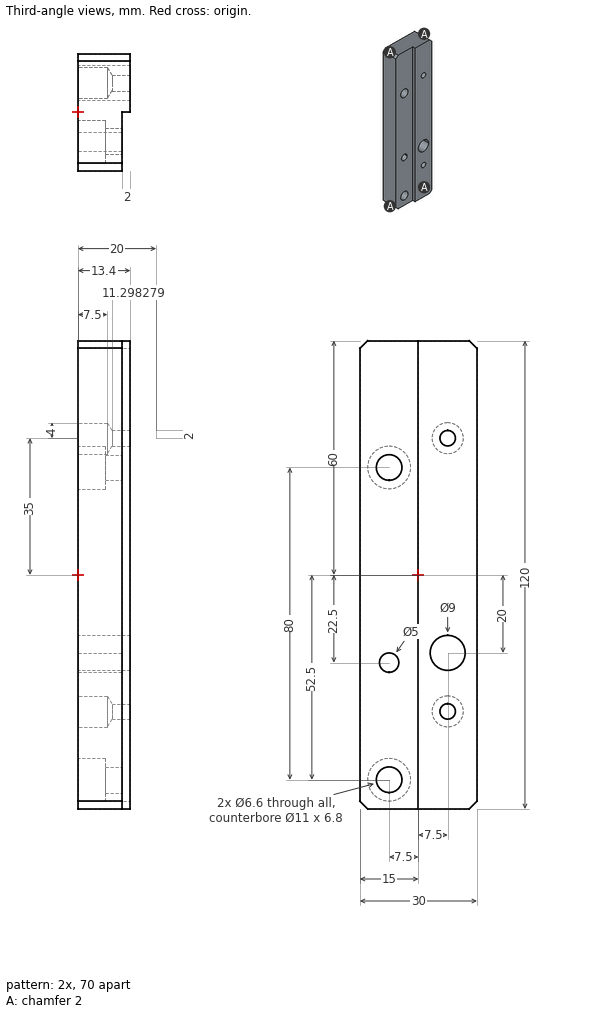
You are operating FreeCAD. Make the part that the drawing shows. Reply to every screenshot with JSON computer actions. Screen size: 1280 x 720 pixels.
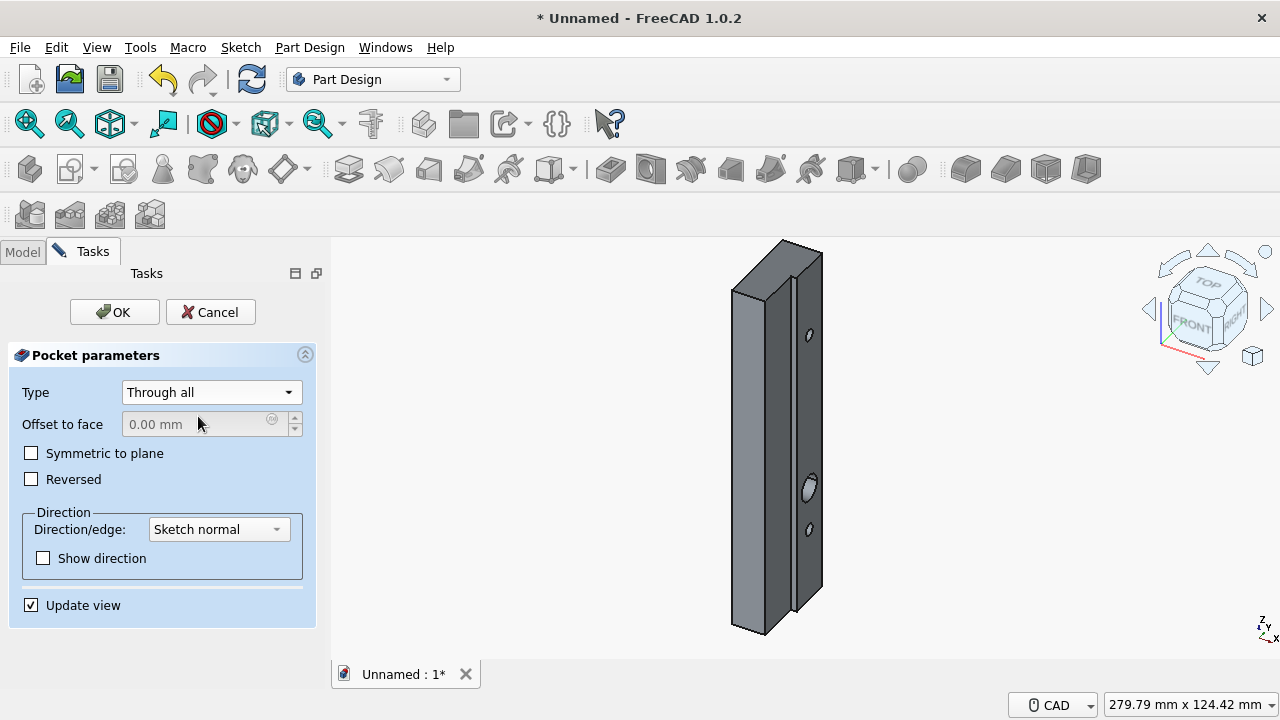
{"action": "left_click", "coordinate": [115, 312]}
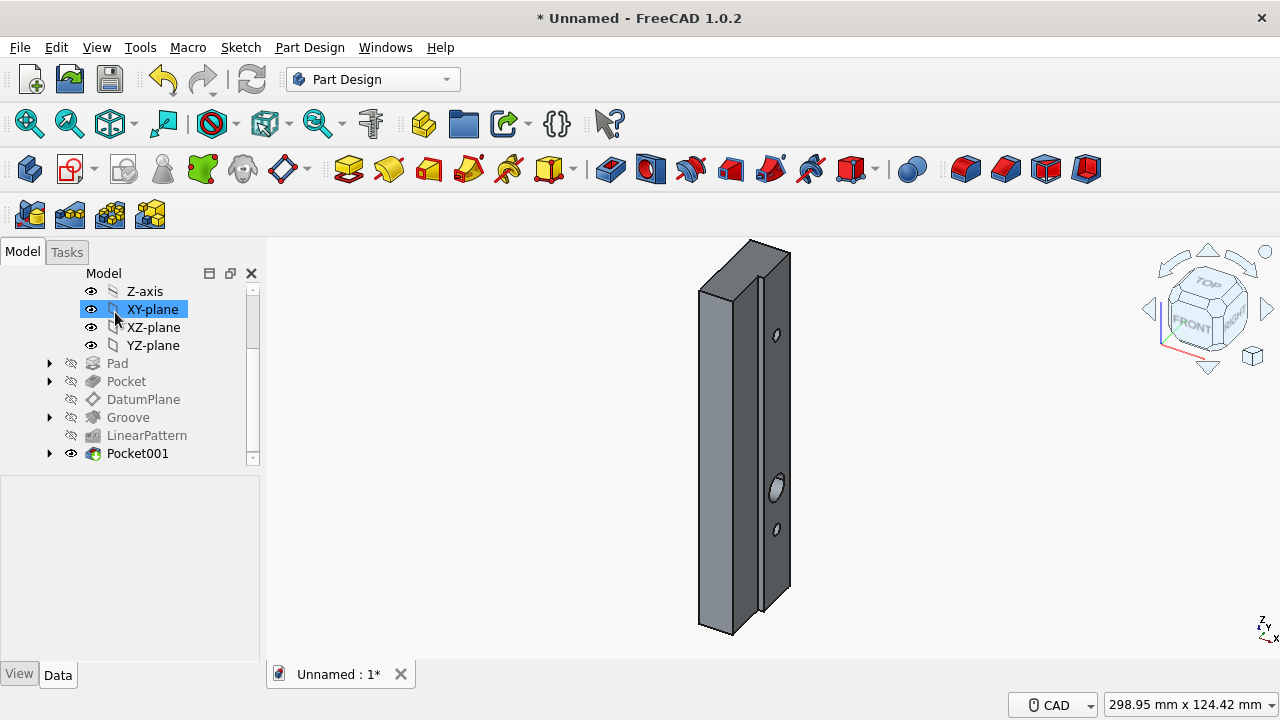
{"action": "left_click", "coordinate": [716, 295]}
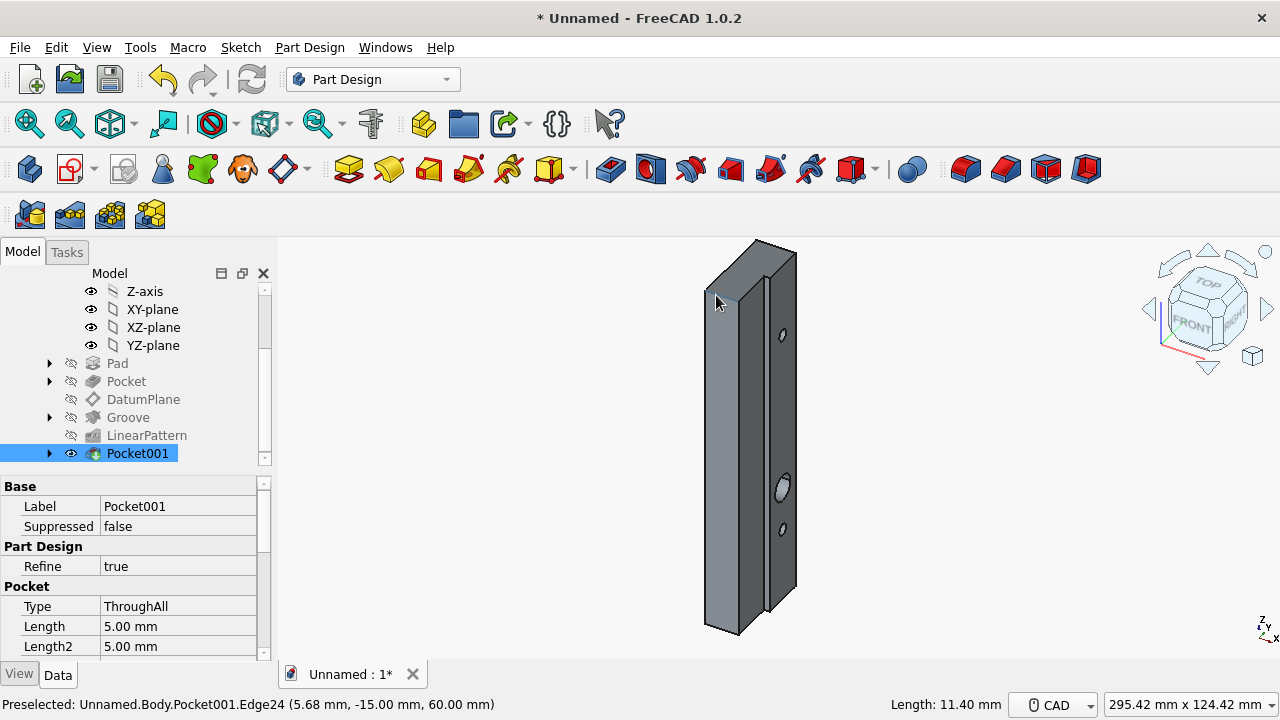
{"action": "key", "text": "0"}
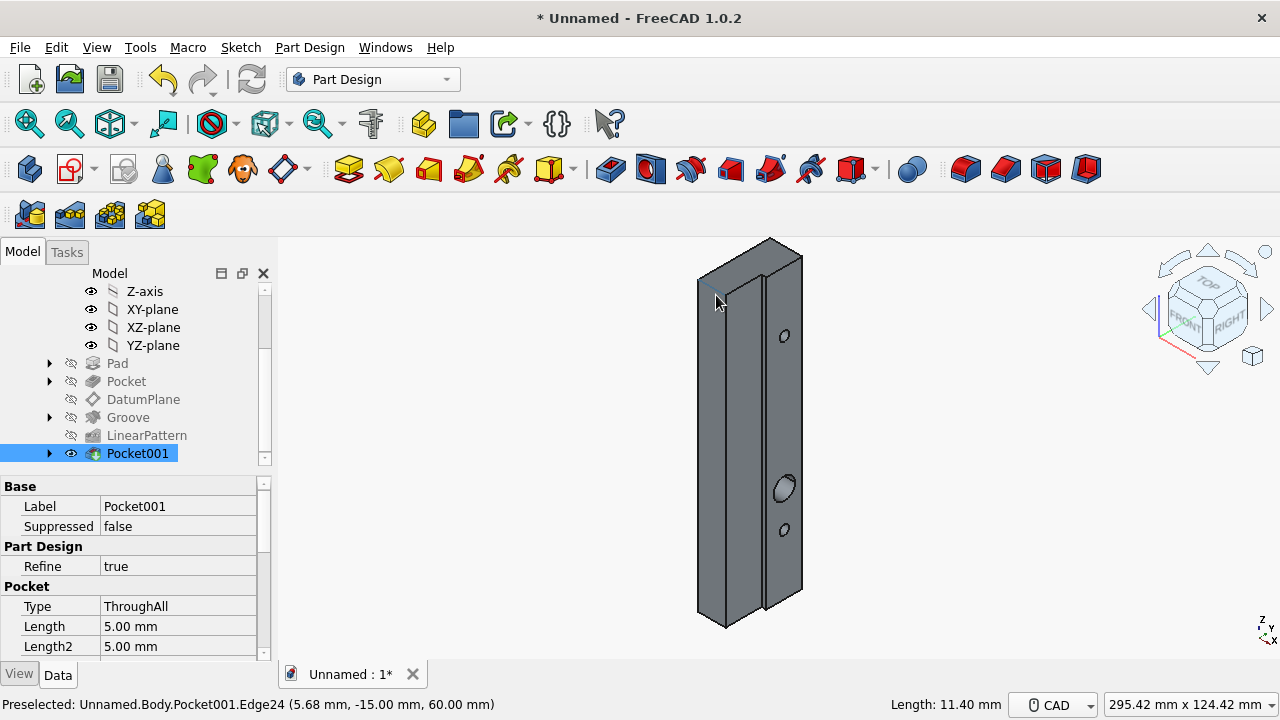
{"action": "key", "text": "2"}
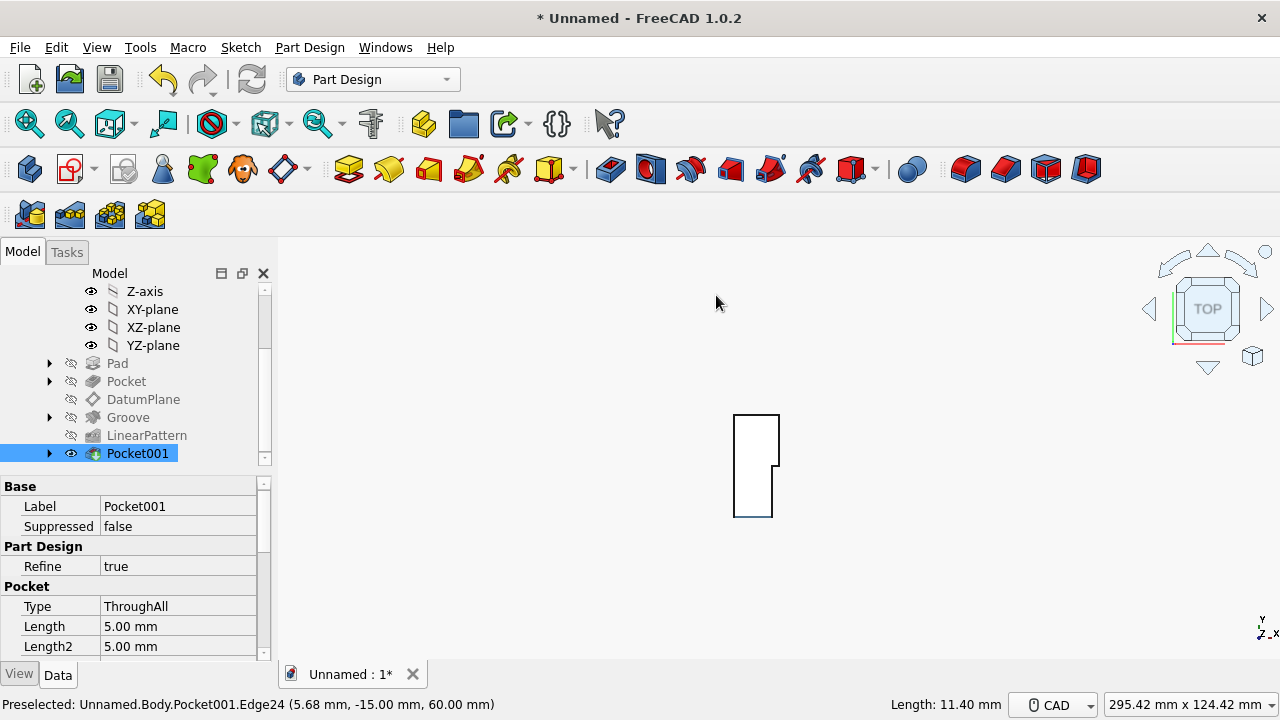
{"action": "left_click", "coordinate": [30, 124]}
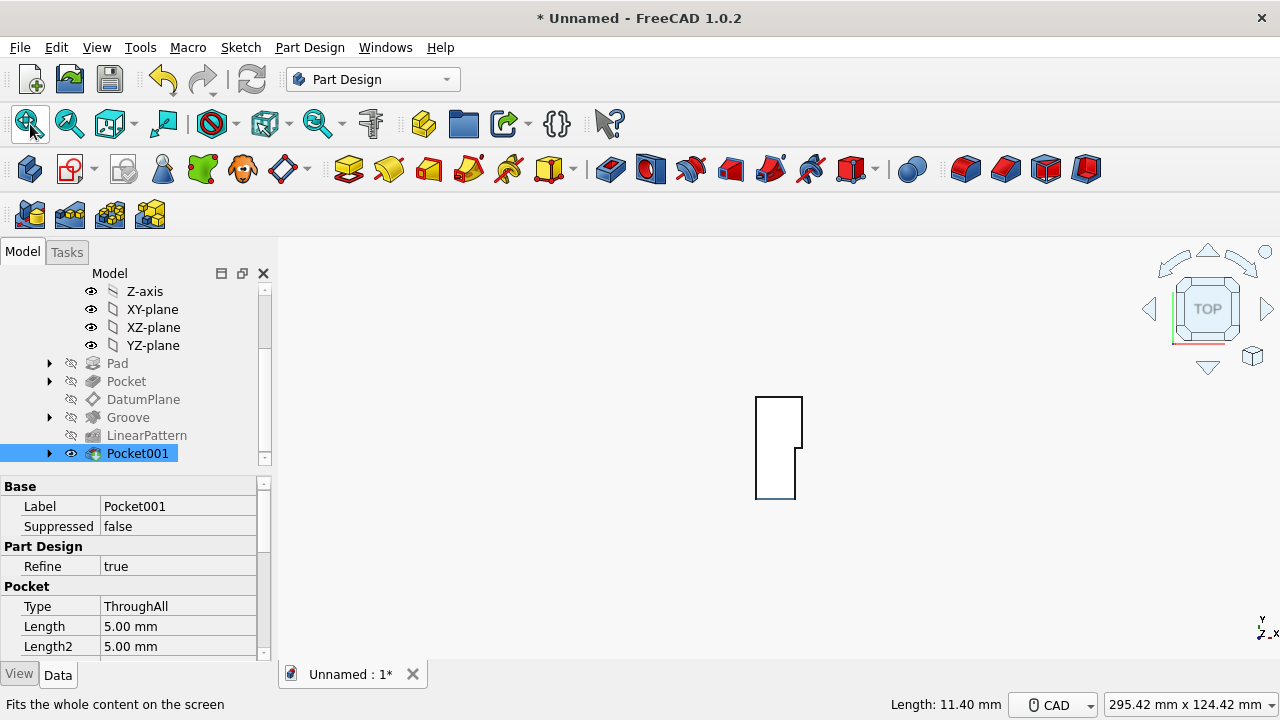
{"action": "left_click", "coordinate": [779, 396], "text": "ctrl"}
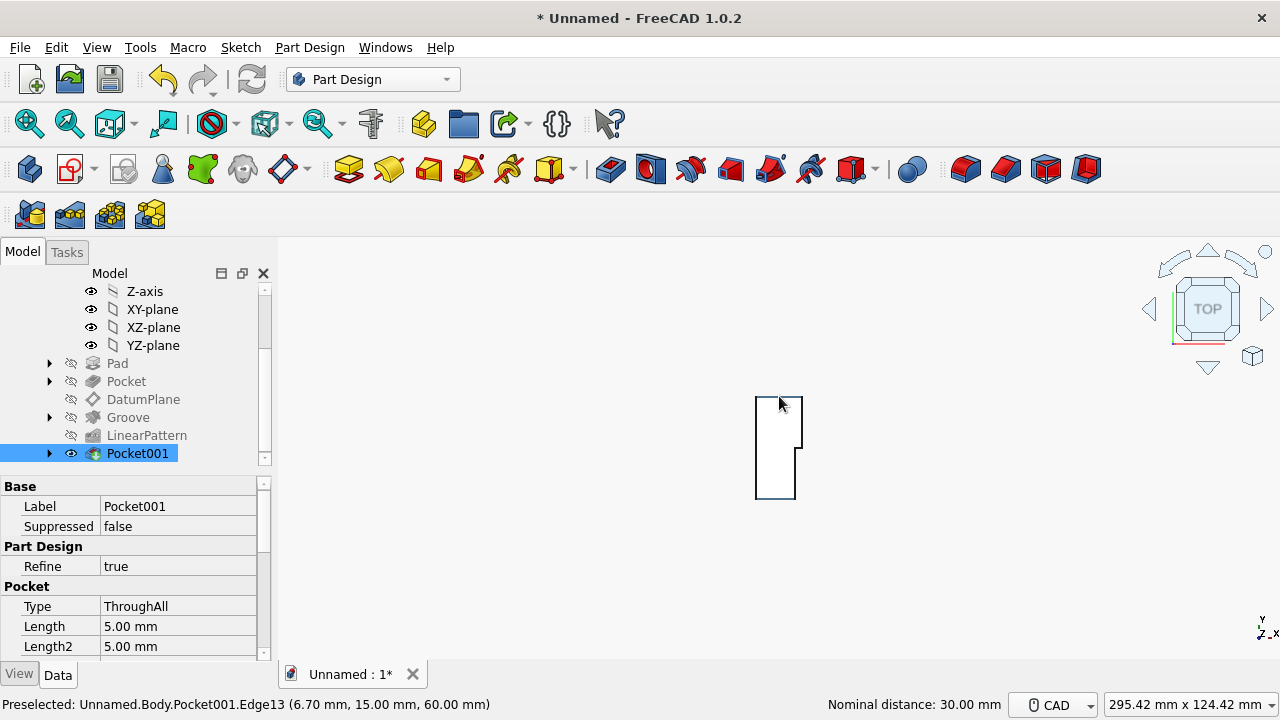
{"action": "key", "text": "1"}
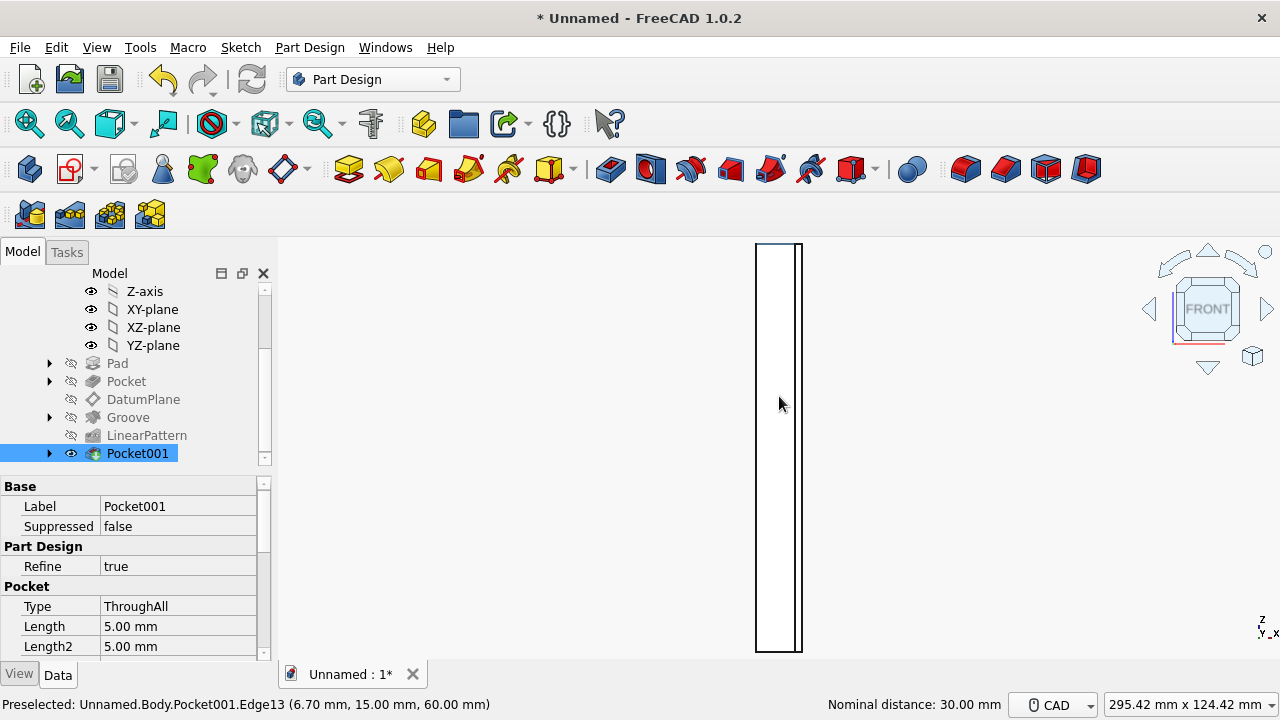
{"action": "key", "text": "3"}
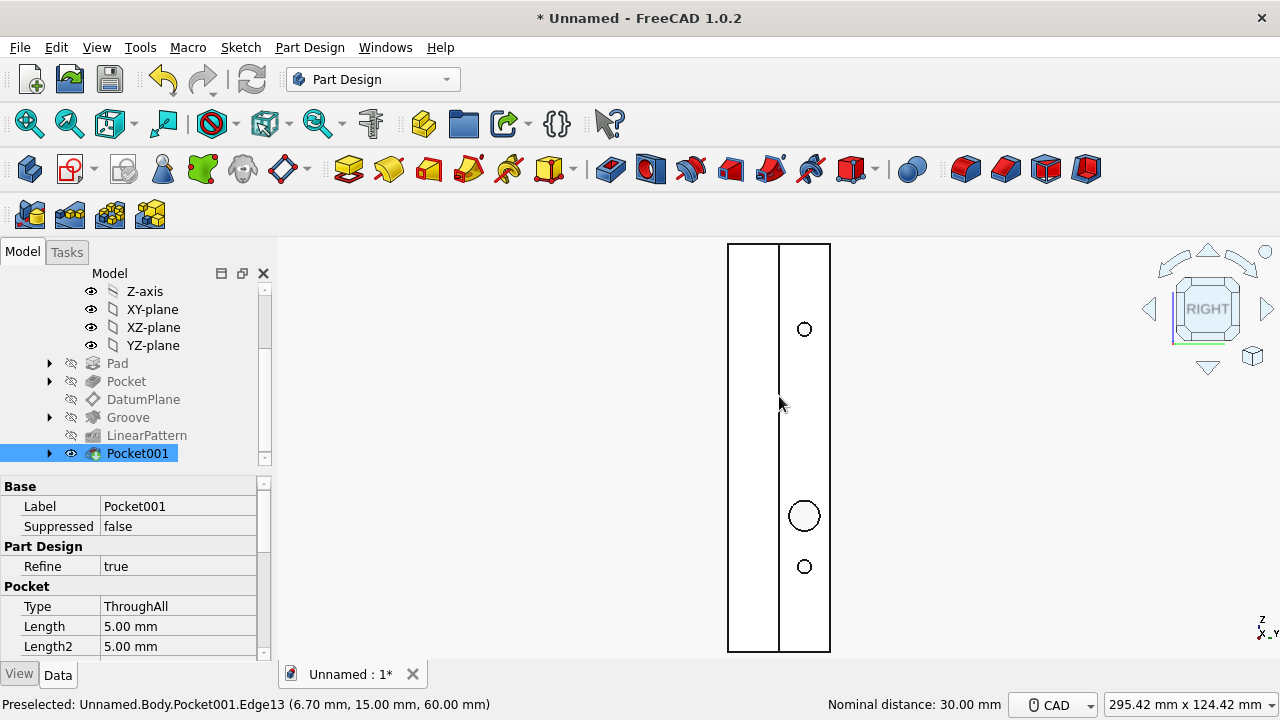
{"action": "key", "text": "5"}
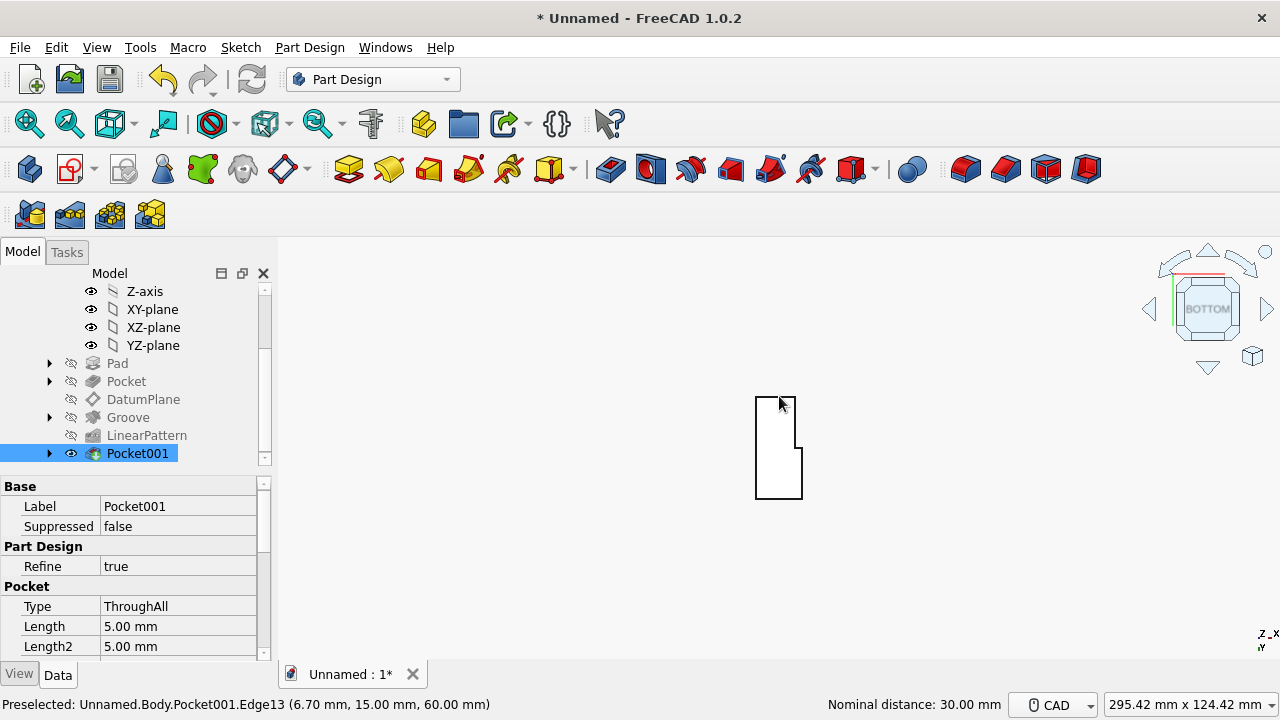
{"action": "left_click", "coordinate": [30, 124]}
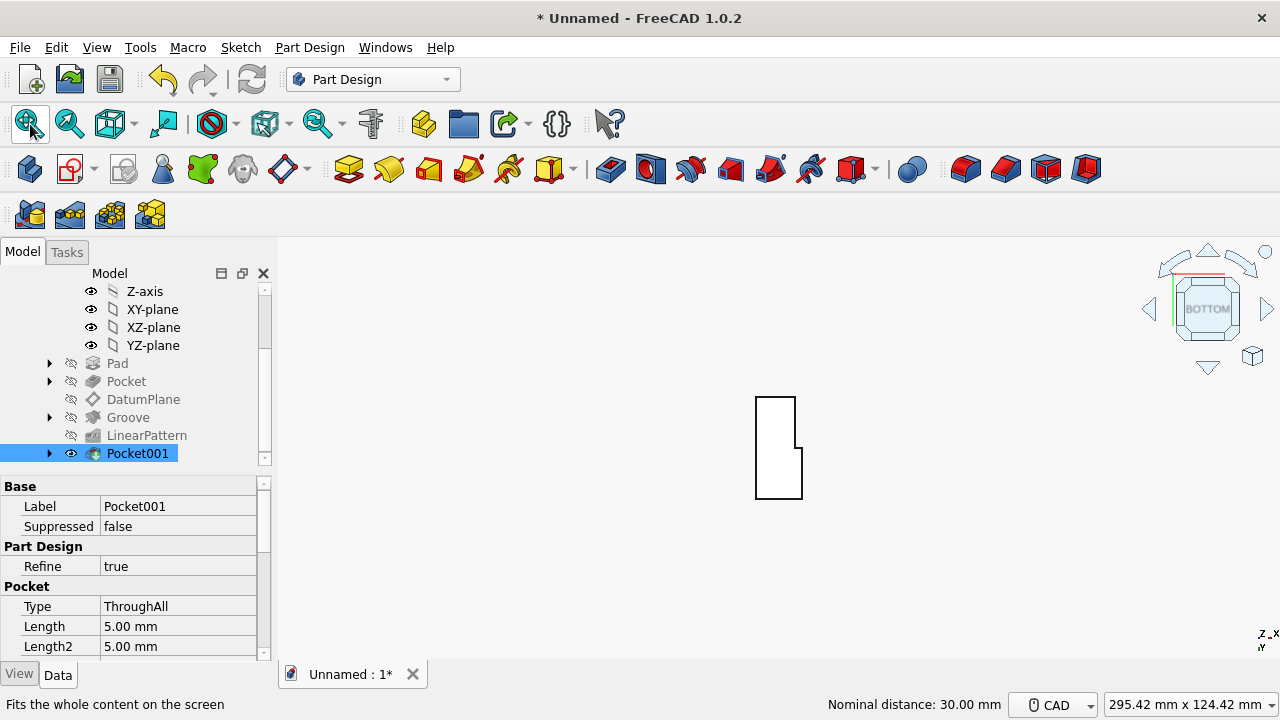
{"action": "left_click", "coordinate": [776, 396], "text": "ctrl"}